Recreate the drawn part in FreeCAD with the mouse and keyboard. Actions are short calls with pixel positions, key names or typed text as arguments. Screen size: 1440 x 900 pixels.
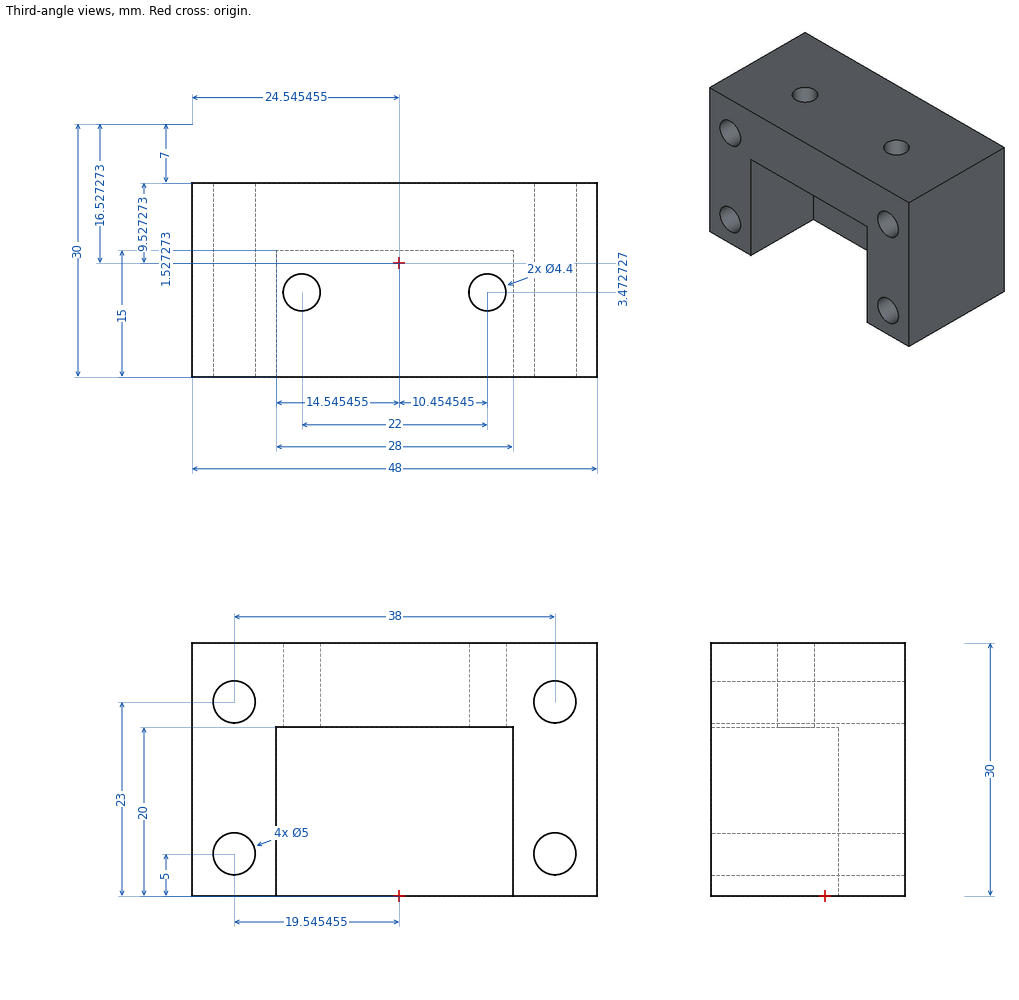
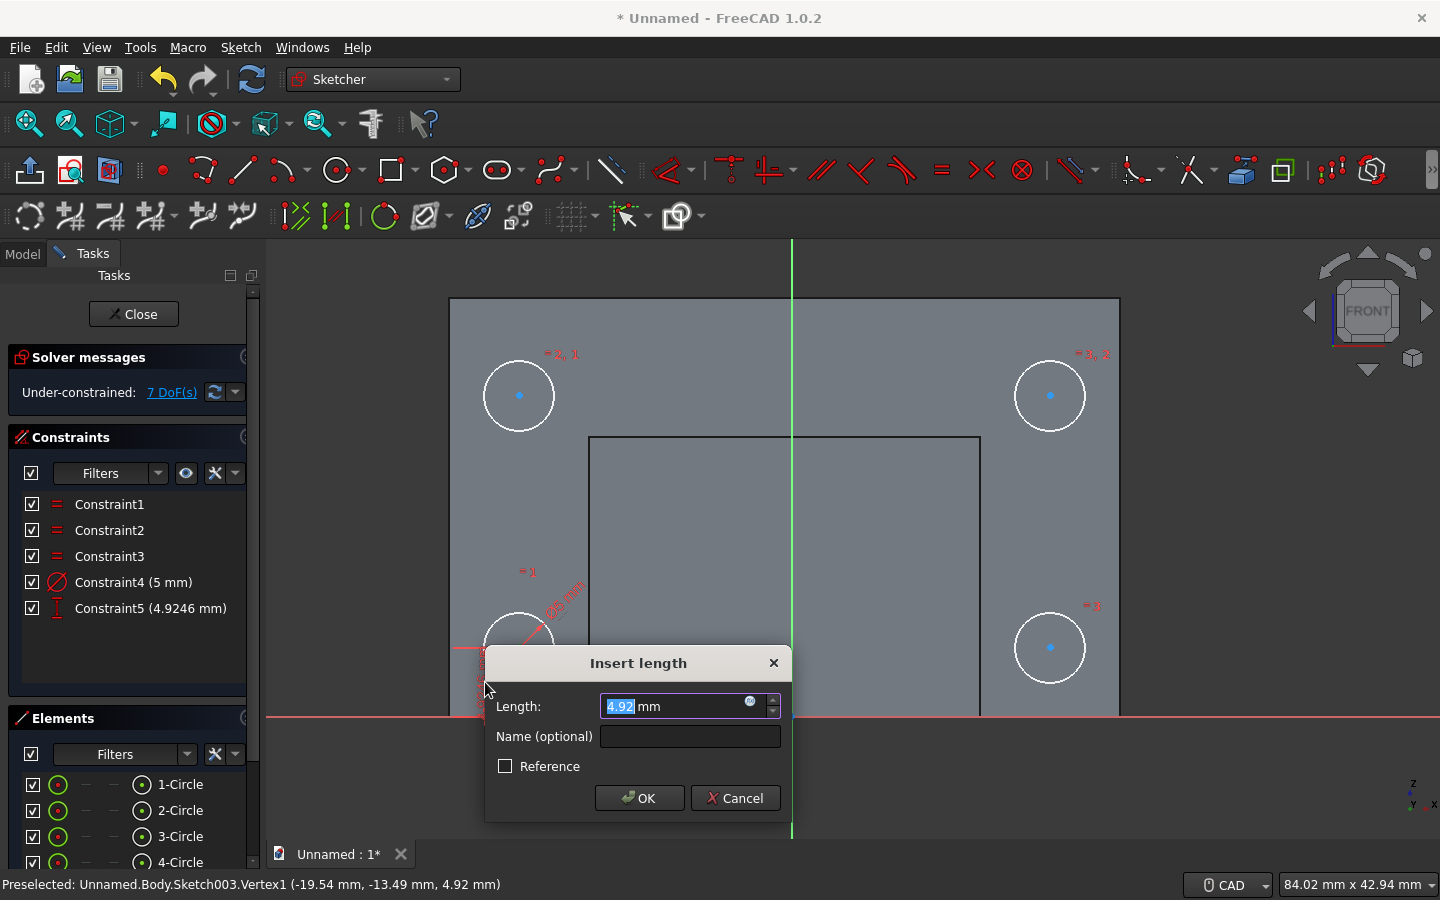
text(5)
key(Return)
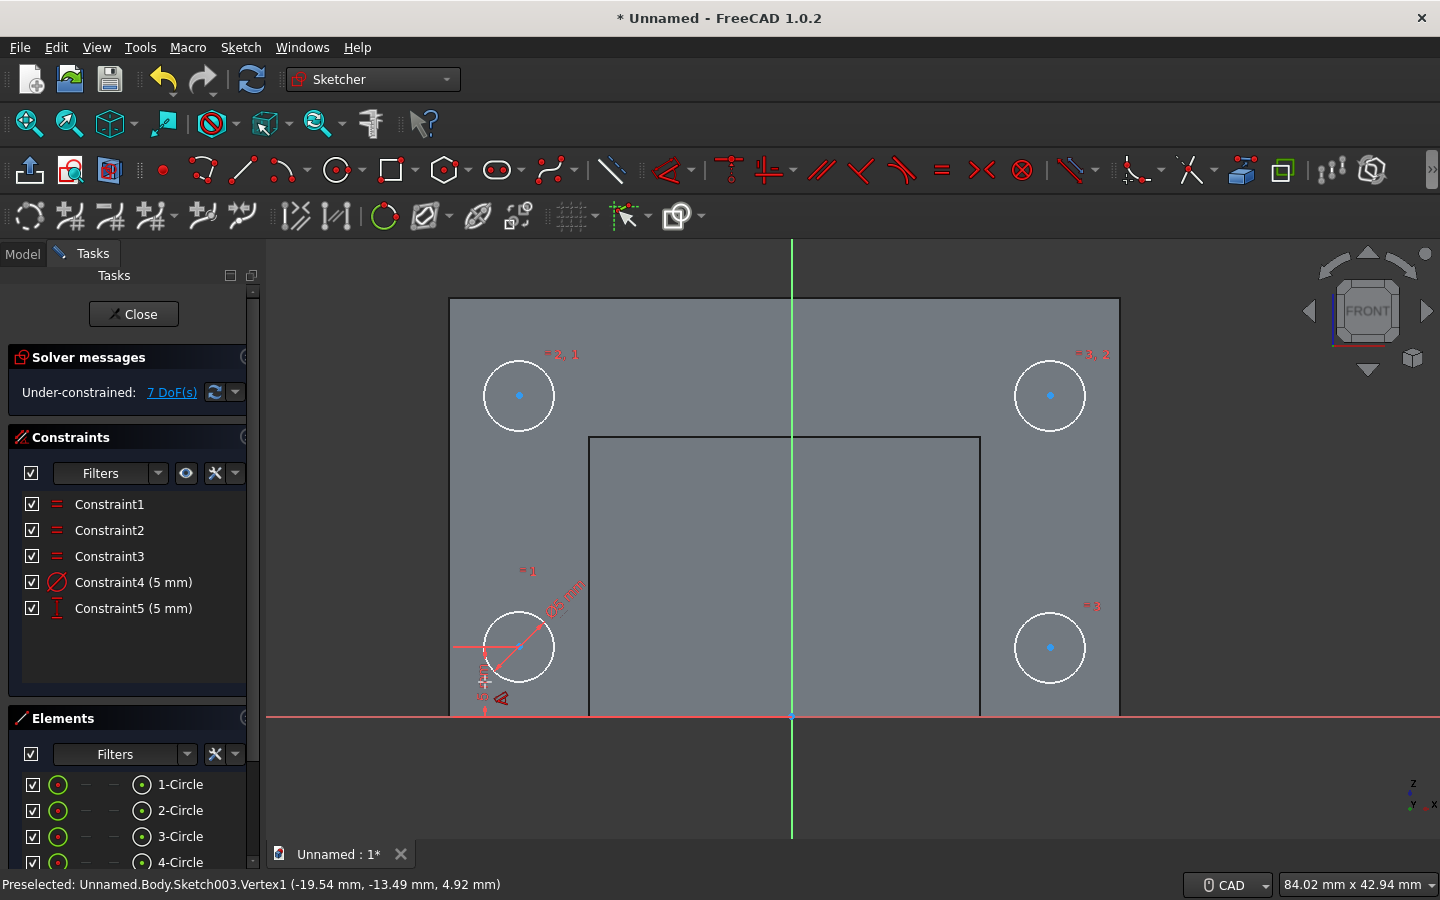
click(1050, 648)
click(1084, 682)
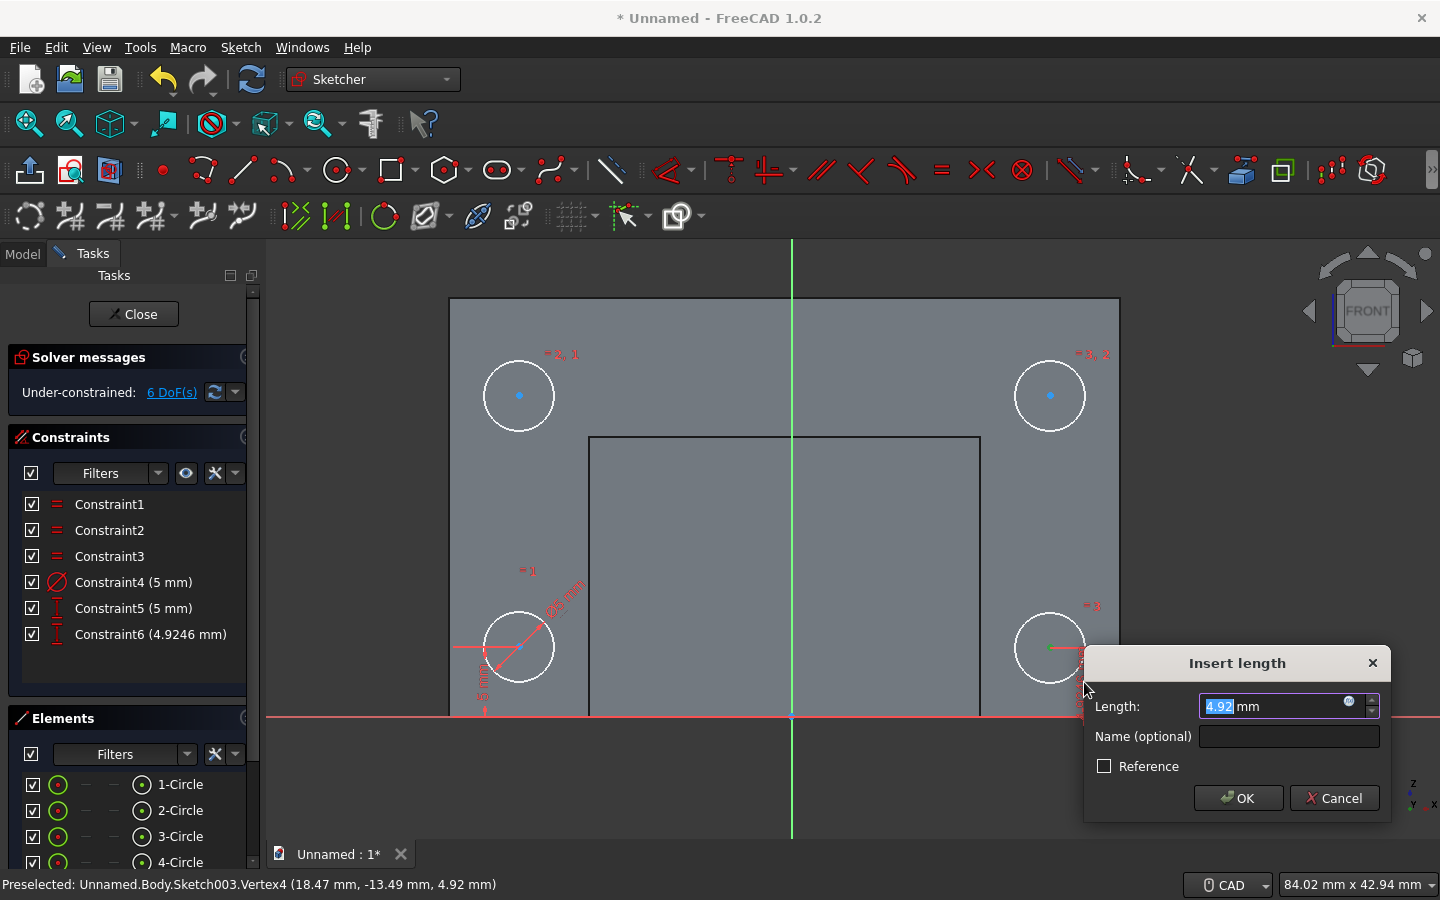
text(5)
key(Return)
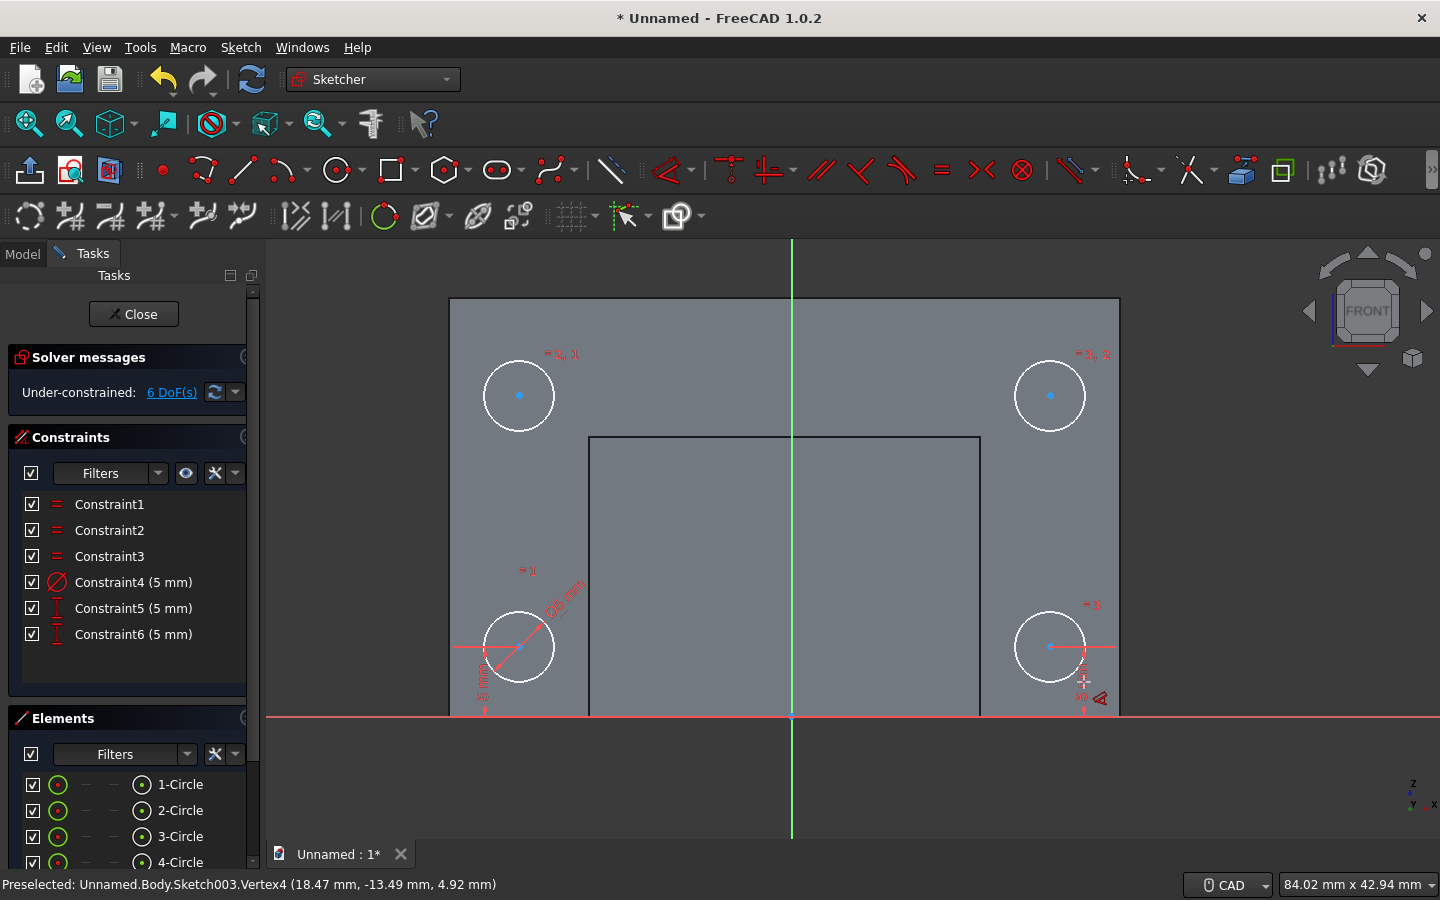
click(519, 396)
click(485, 556)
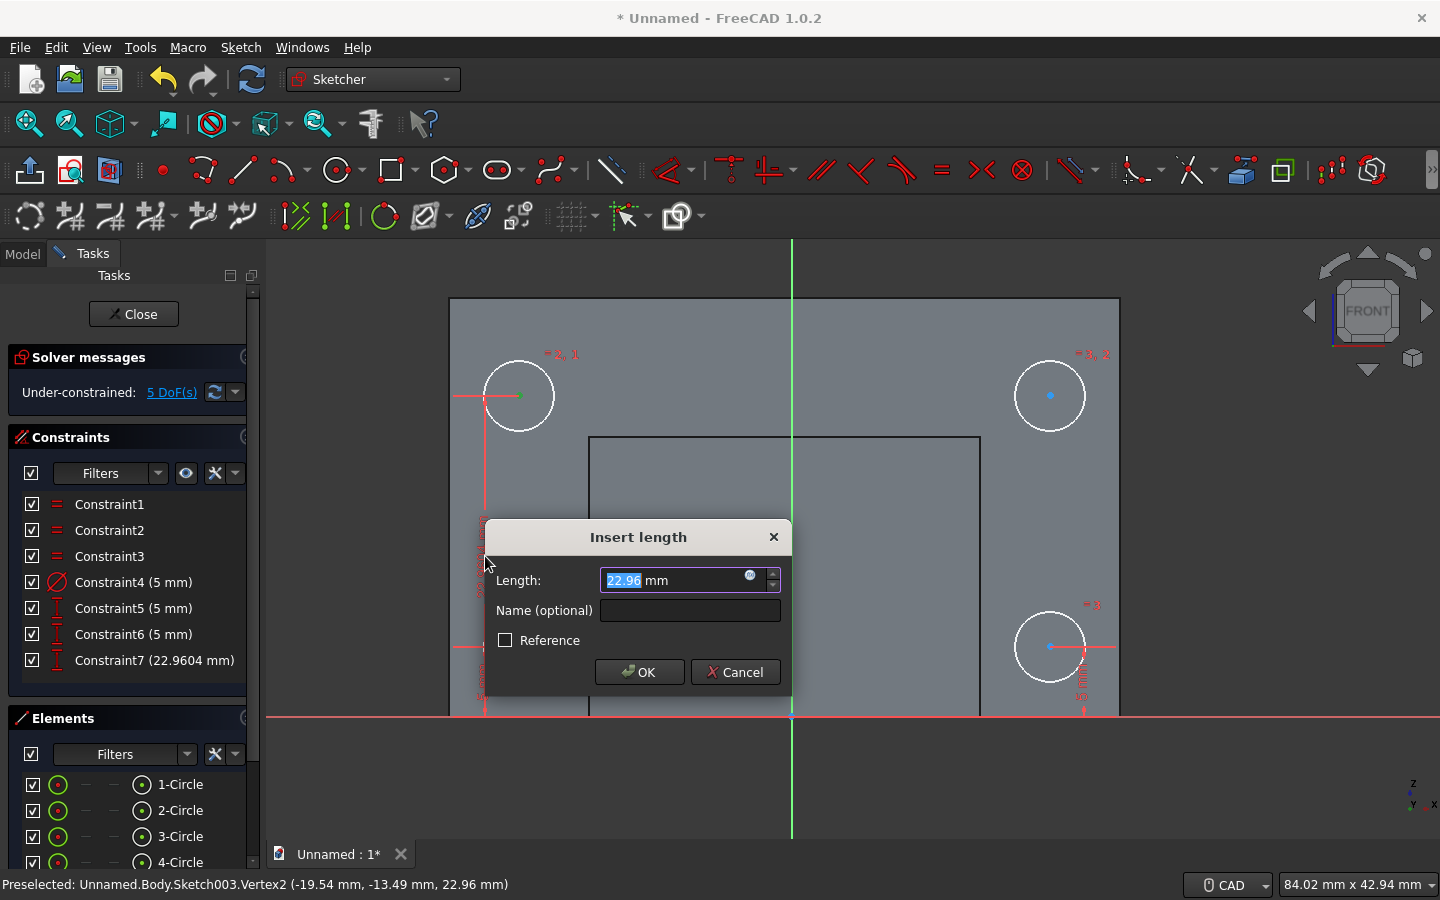
text(23)
key(Return)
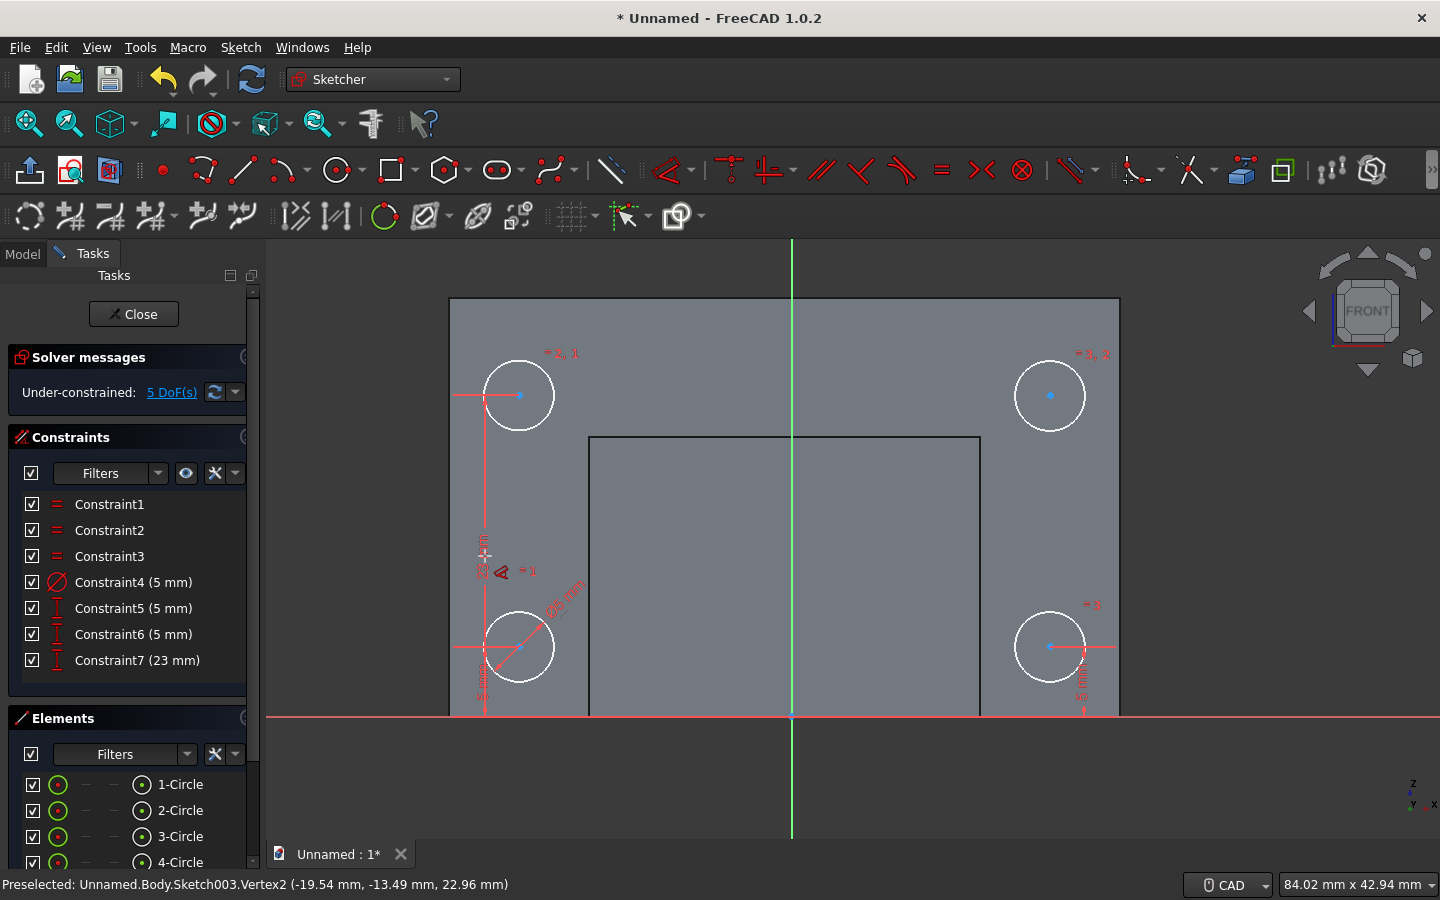
click(1050, 396)
click(1084, 556)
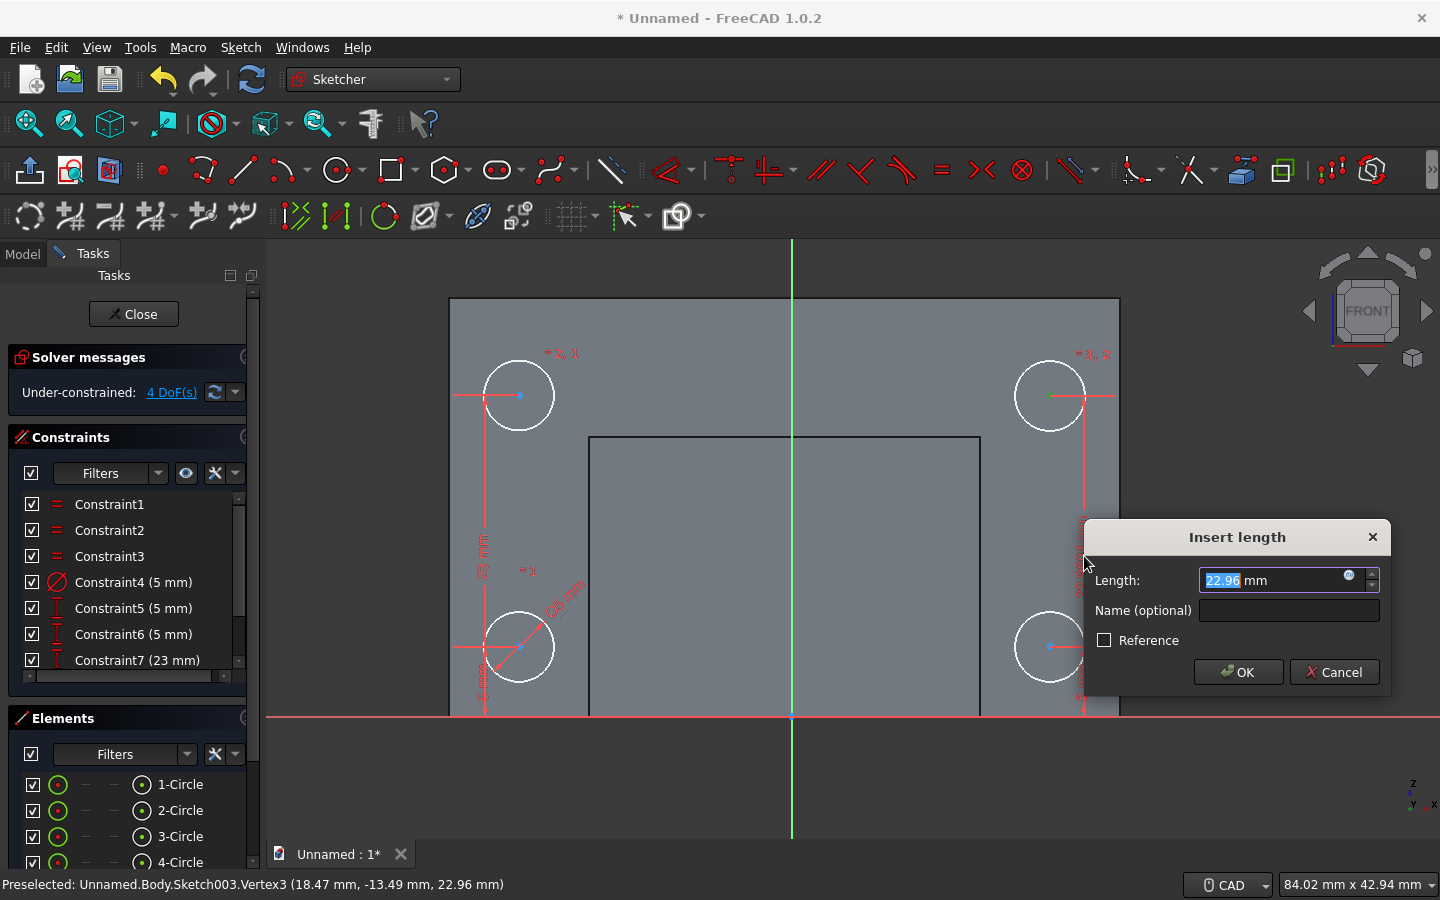
text(23)
key(Return)